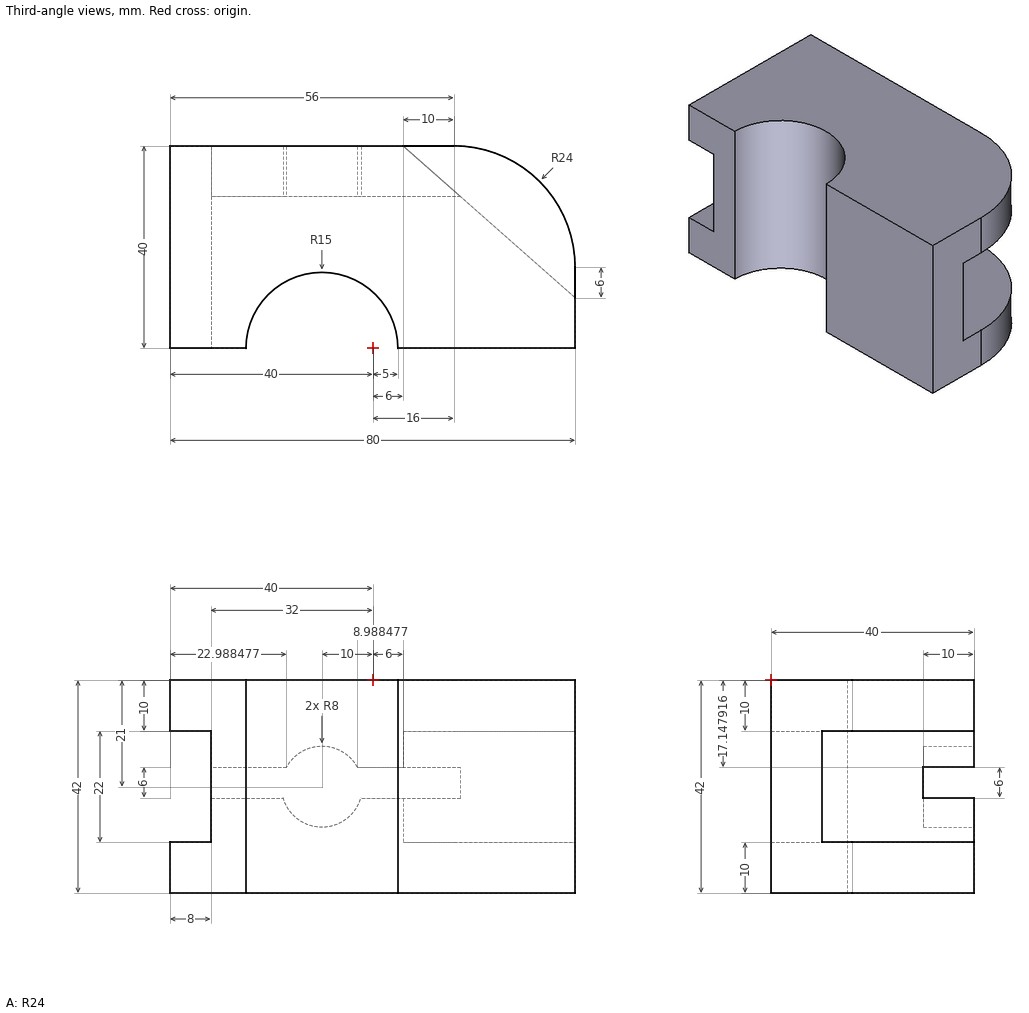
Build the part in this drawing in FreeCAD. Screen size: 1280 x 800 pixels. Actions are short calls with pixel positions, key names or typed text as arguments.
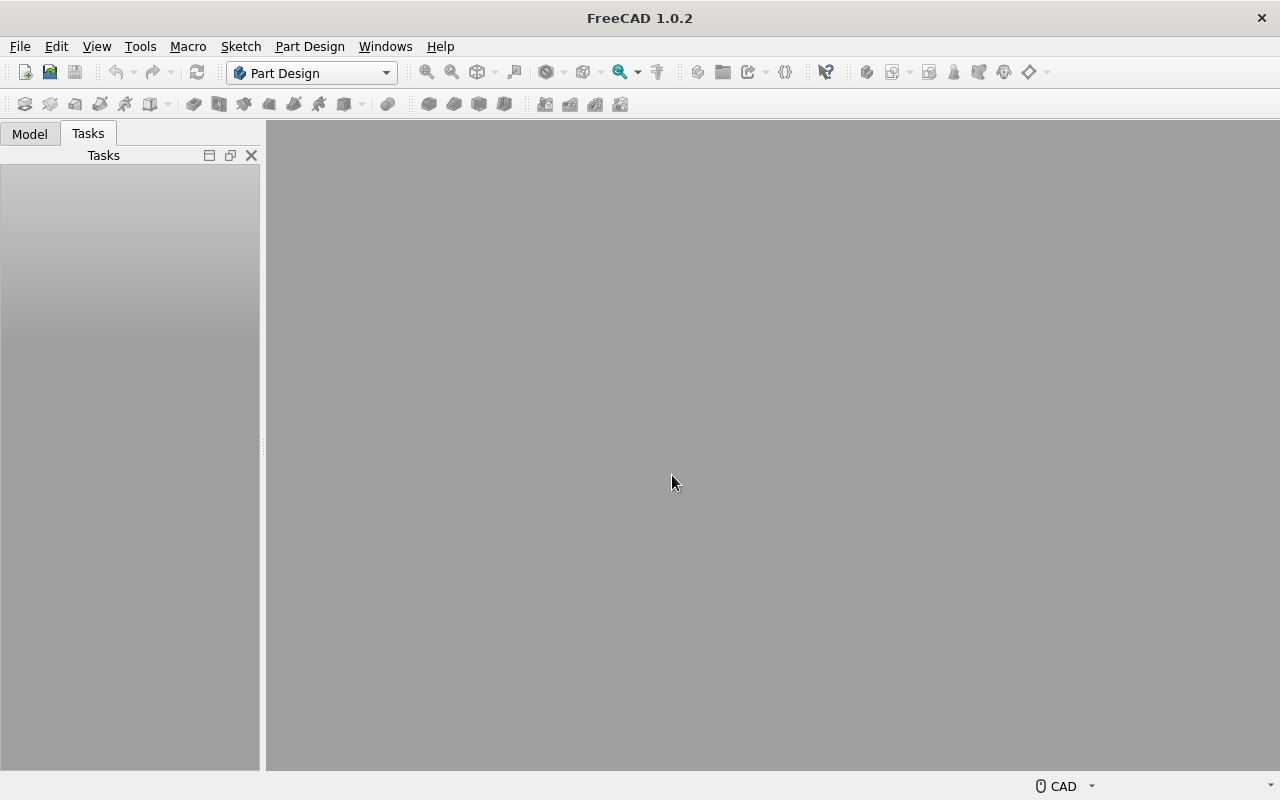
click(25, 72)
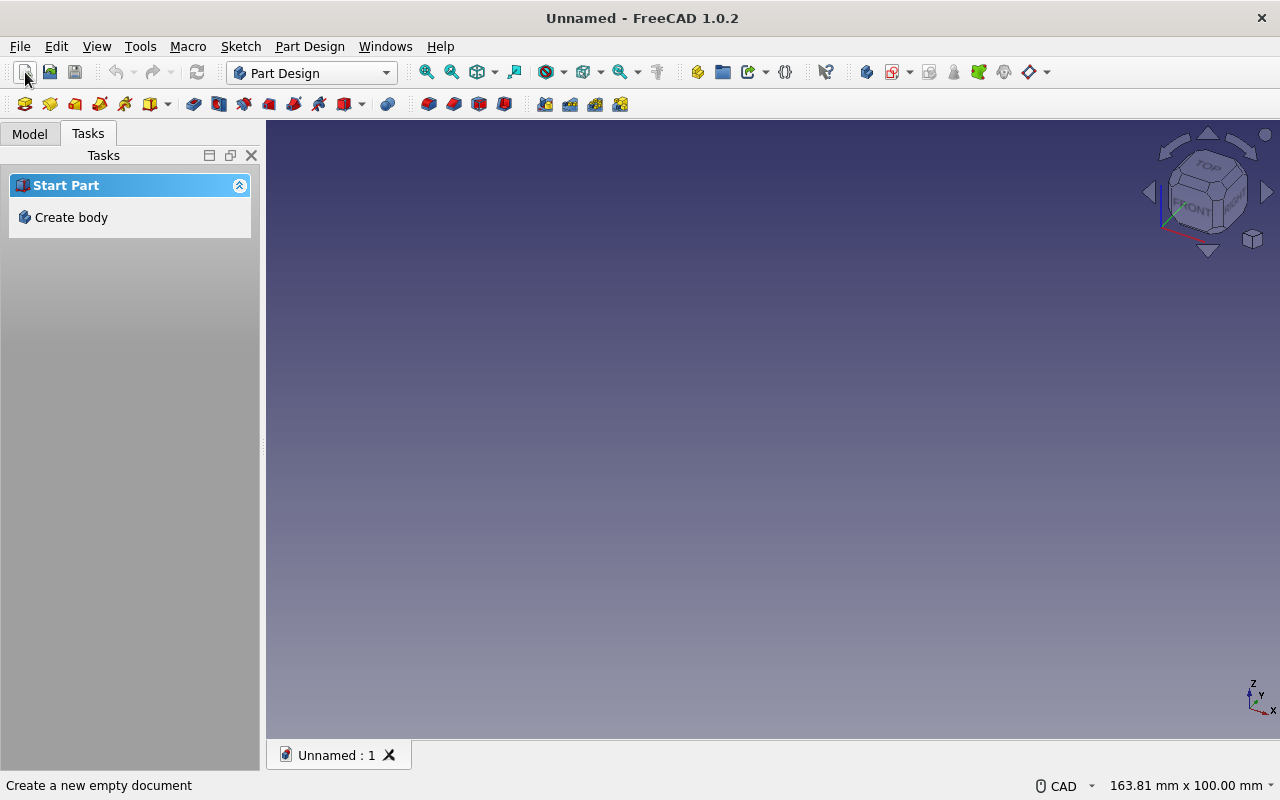
click(892, 72)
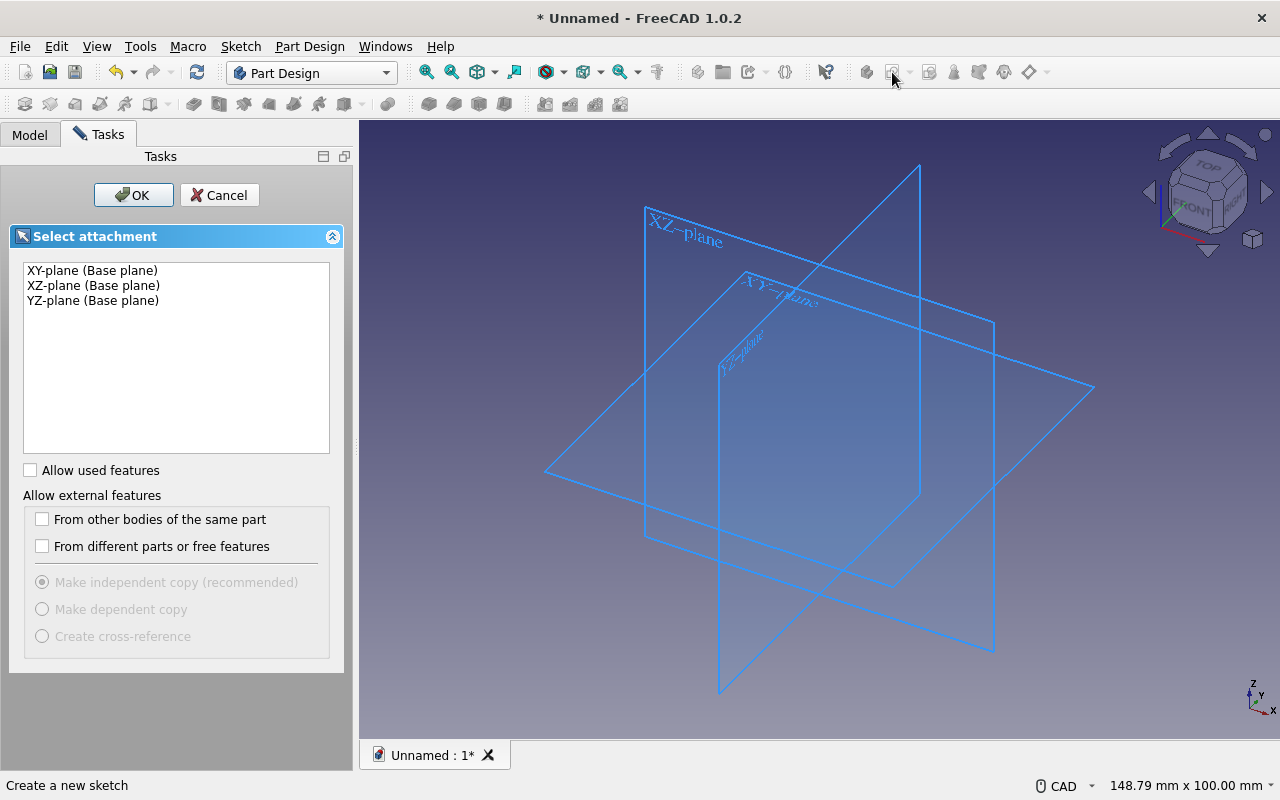
click(84, 270)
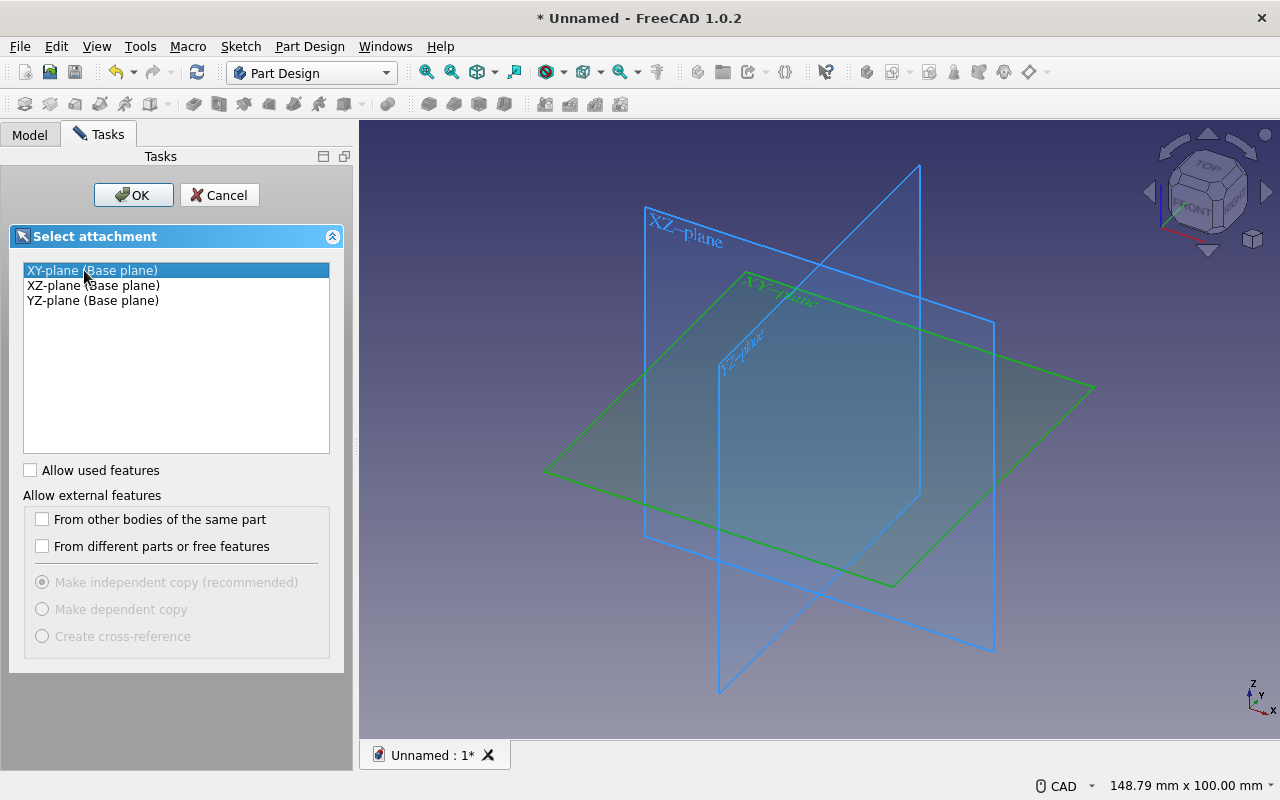
click(134, 195)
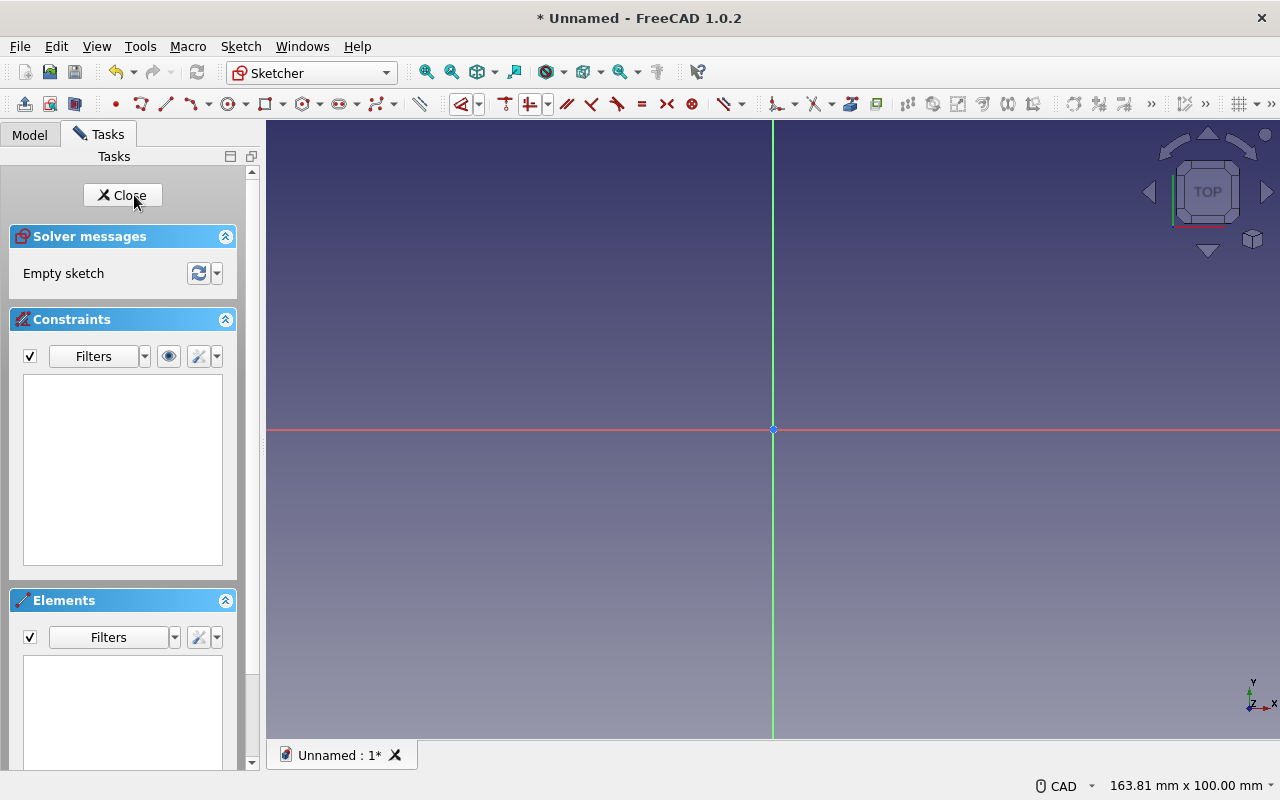
click(141, 104)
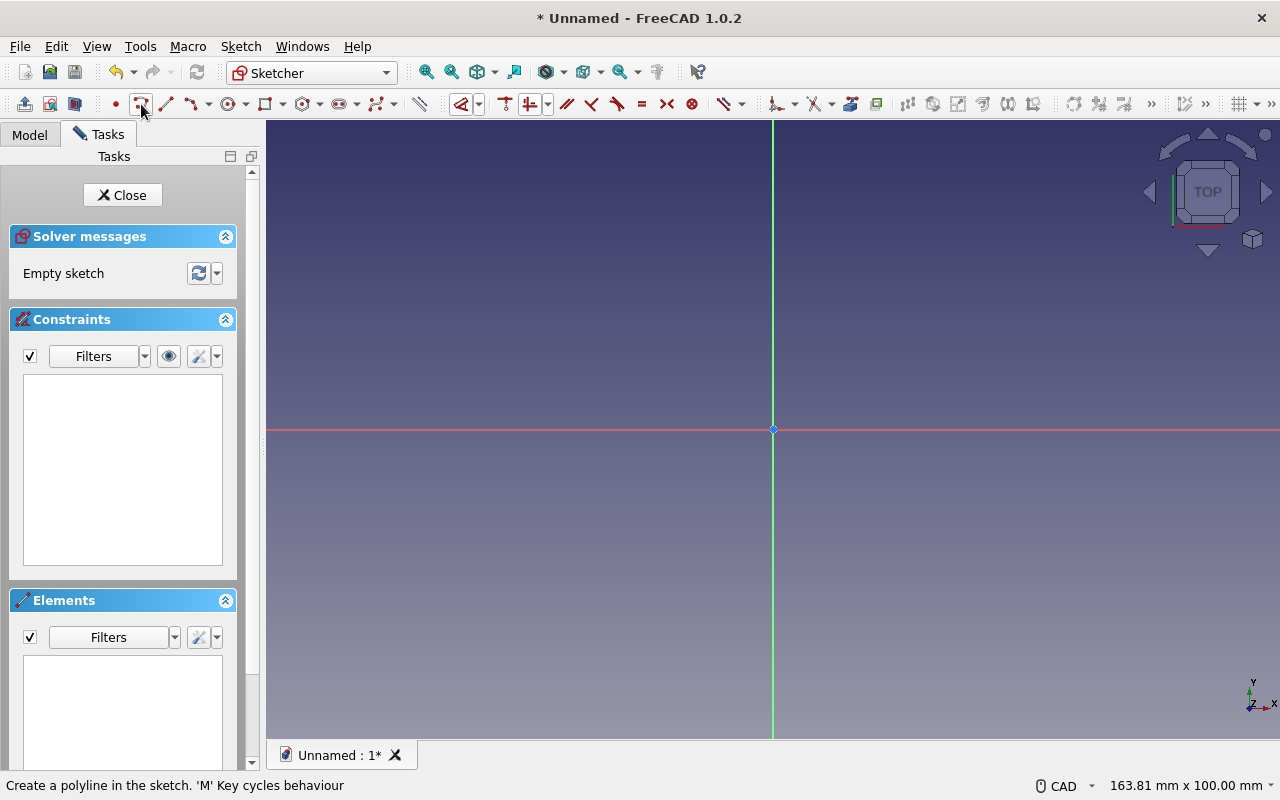
click(872, 182)
click(525, 182)
click(525, 430)
click(1021, 420)
click(1021, 330)
right_click(1021, 330)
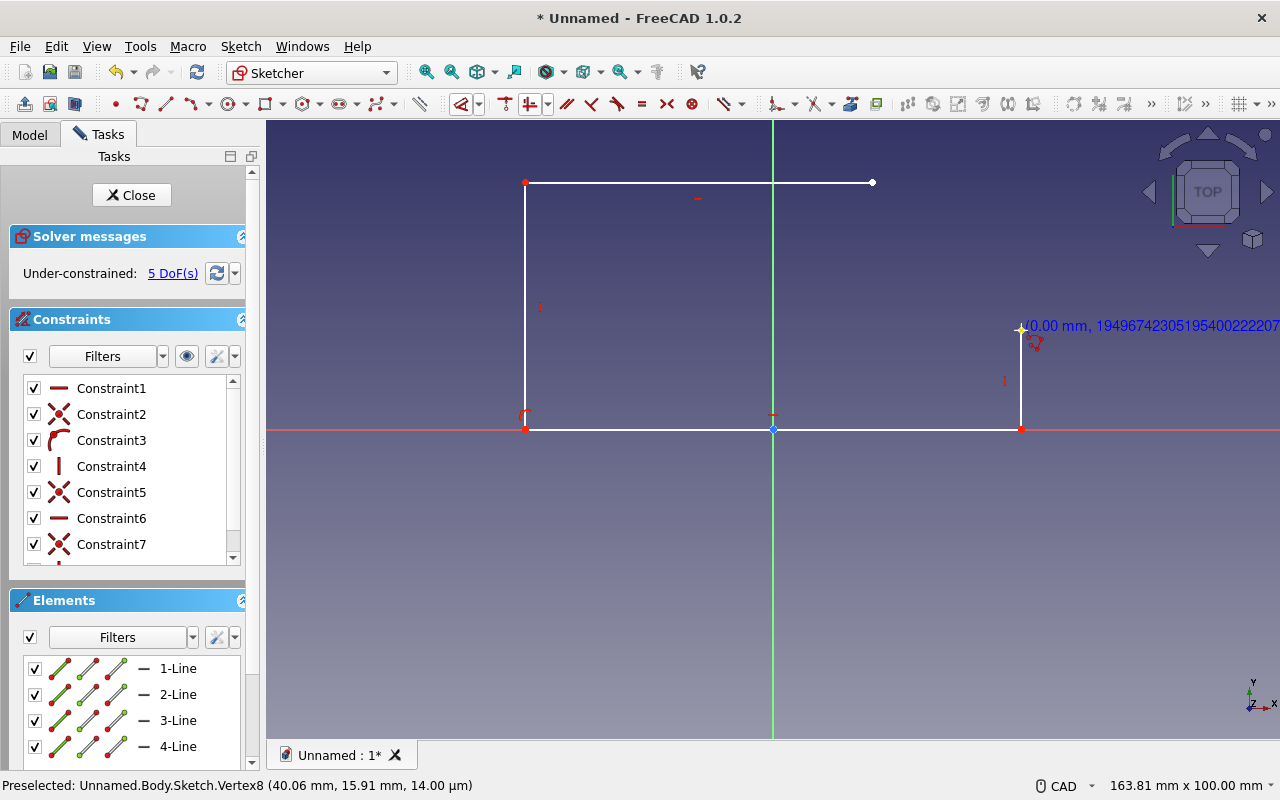
click(190, 104)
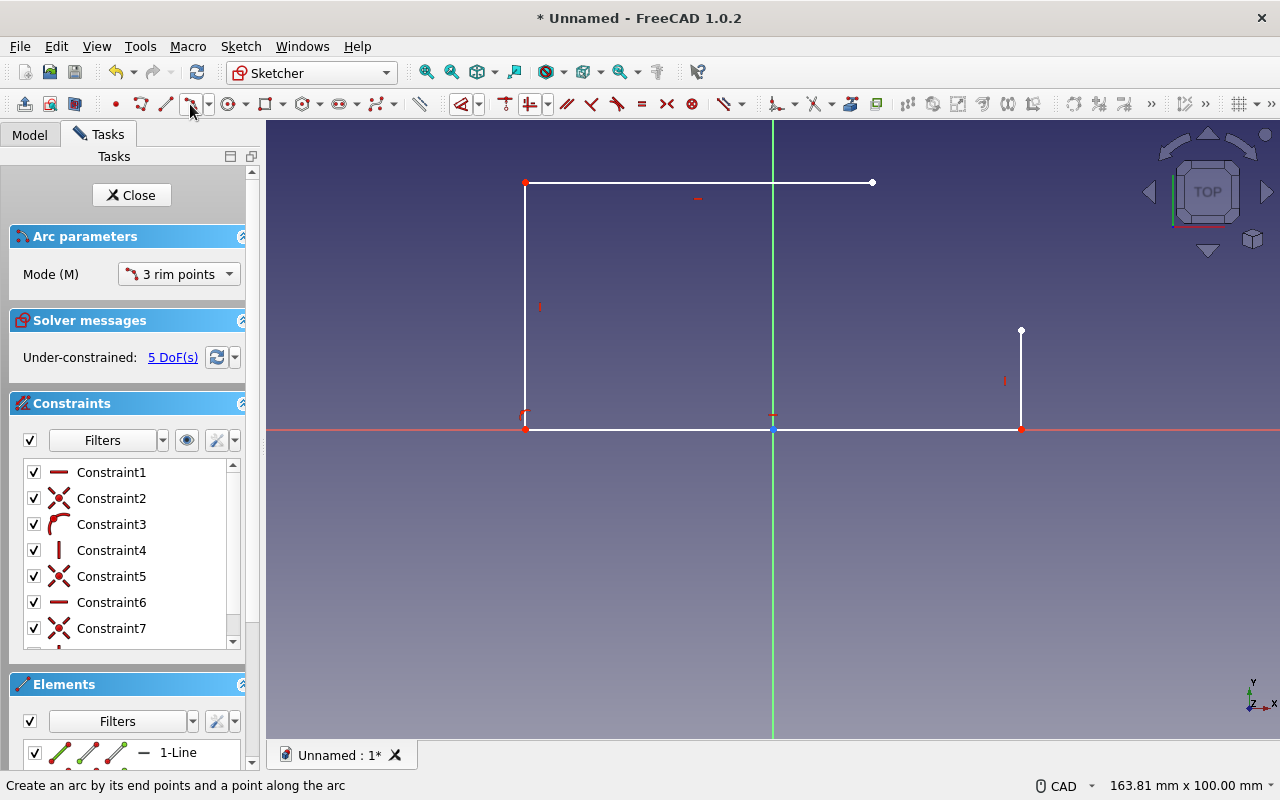
click(1021, 331)
click(872, 183)
click(977, 225)
key(Escape)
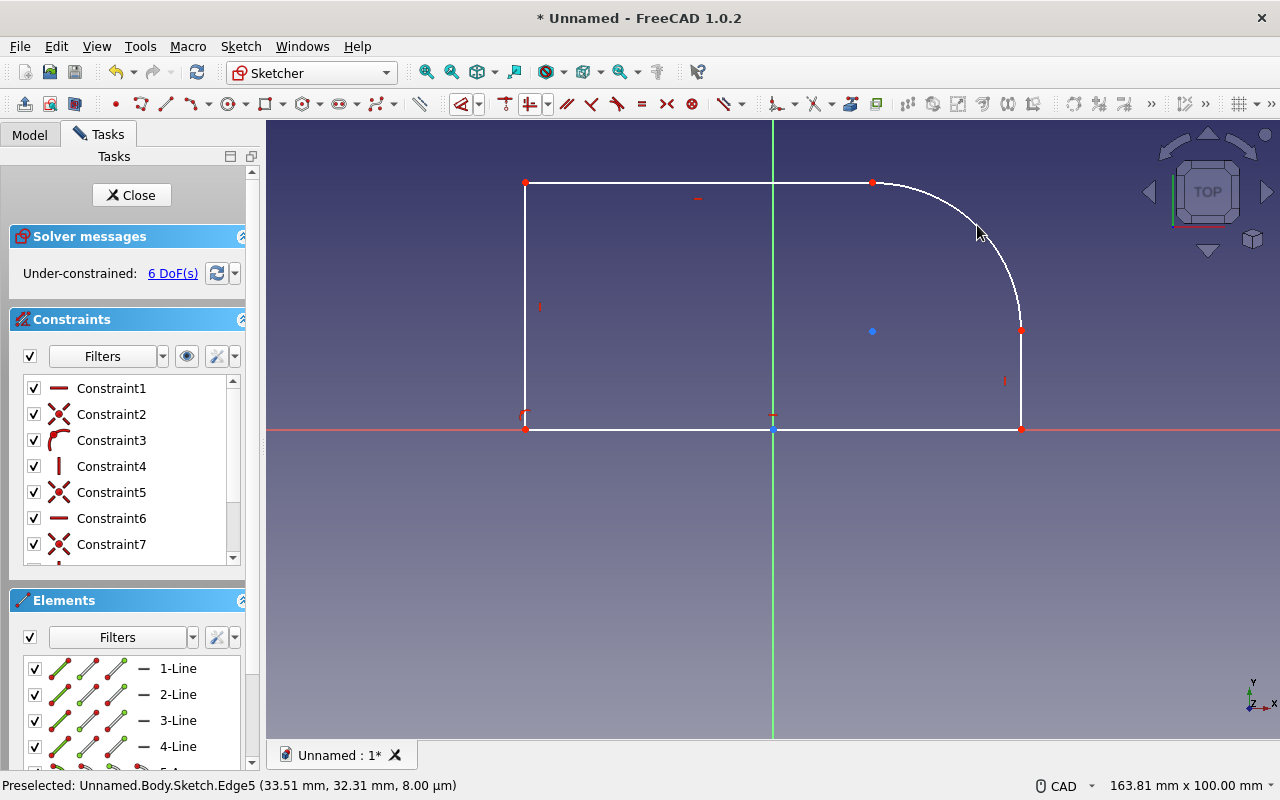
click(629, 183)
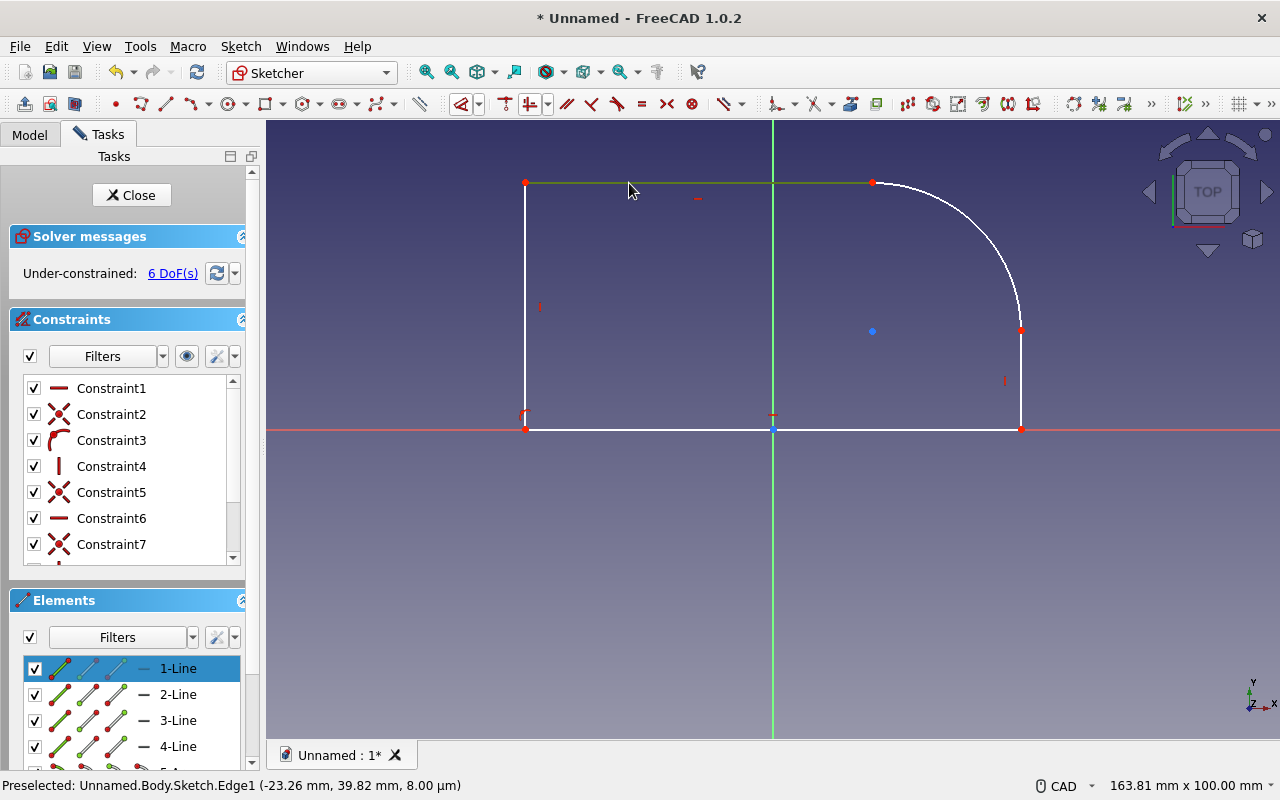
click(1005, 264)